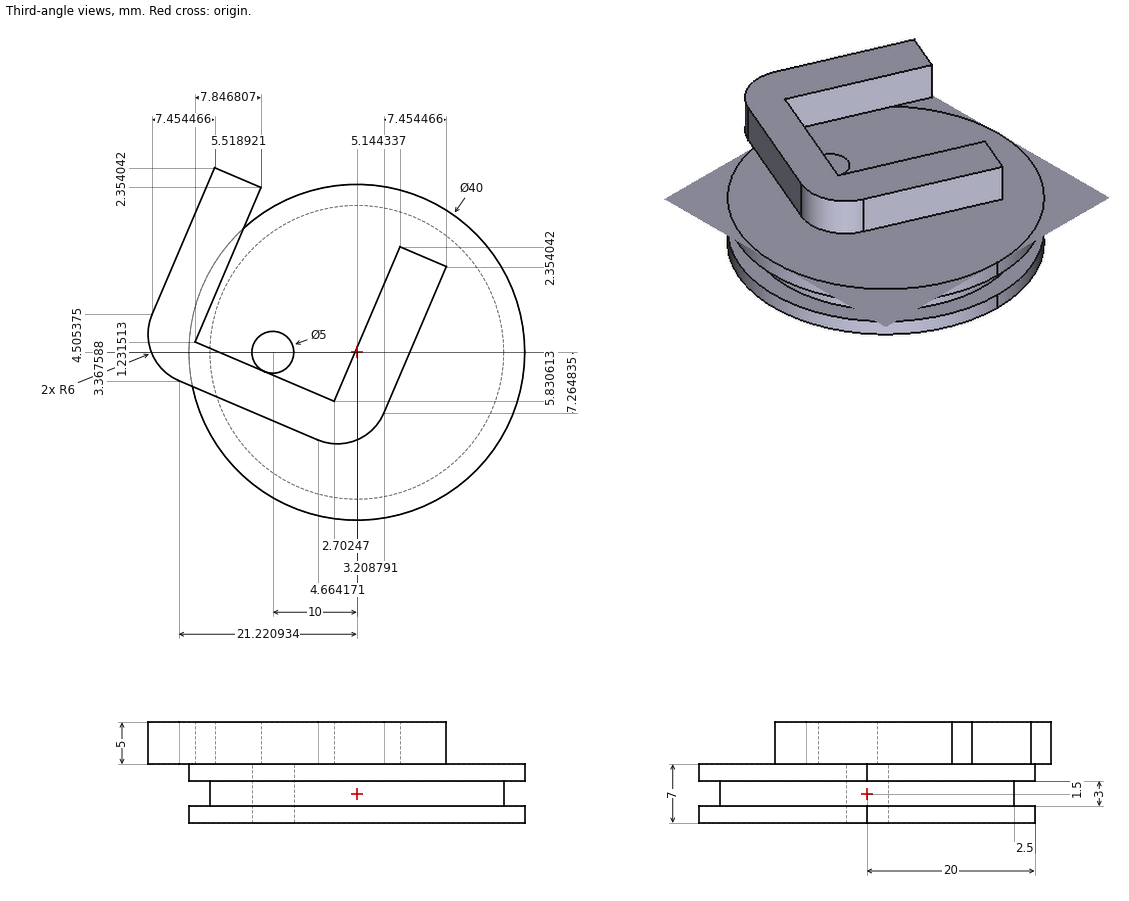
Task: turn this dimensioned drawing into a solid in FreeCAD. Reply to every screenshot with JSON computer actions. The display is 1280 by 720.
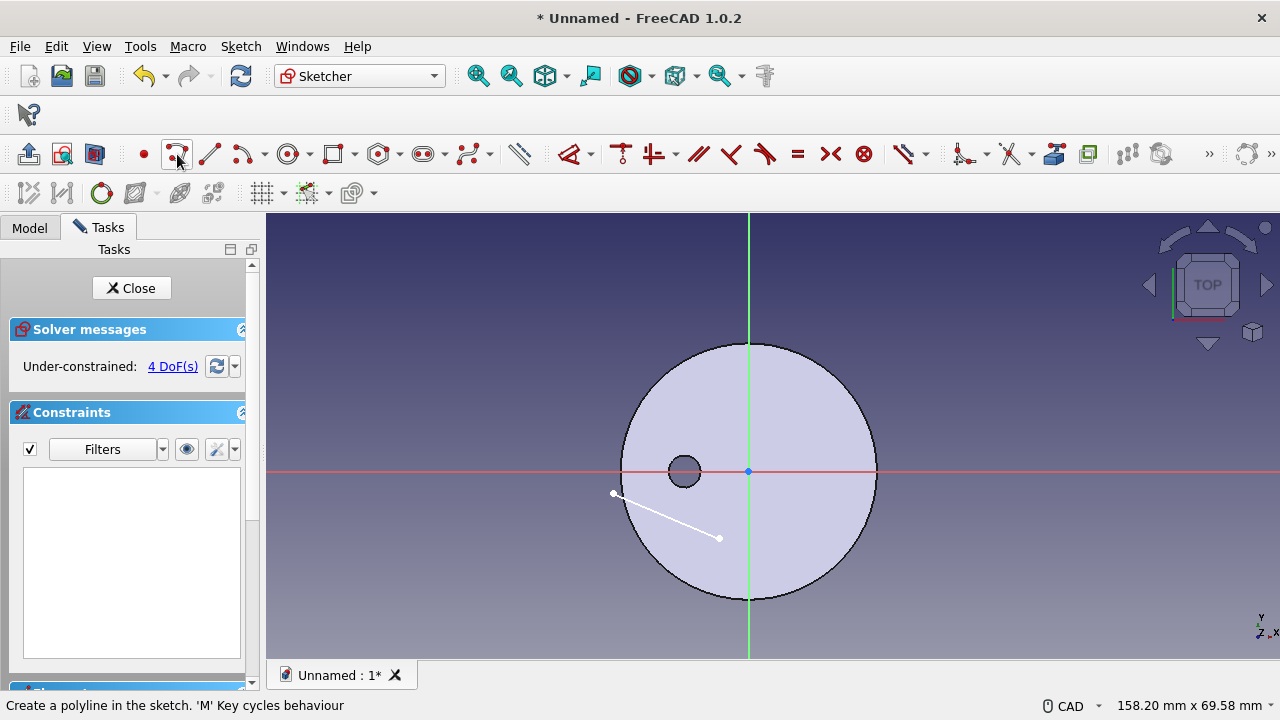
{"action": "left_click", "coordinate": [769, 518]}
{"action": "left_click", "coordinate": [817, 406]}
{"action": "left_click", "coordinate": [782, 391]}
{"action": "left_click", "coordinate": [731, 509]}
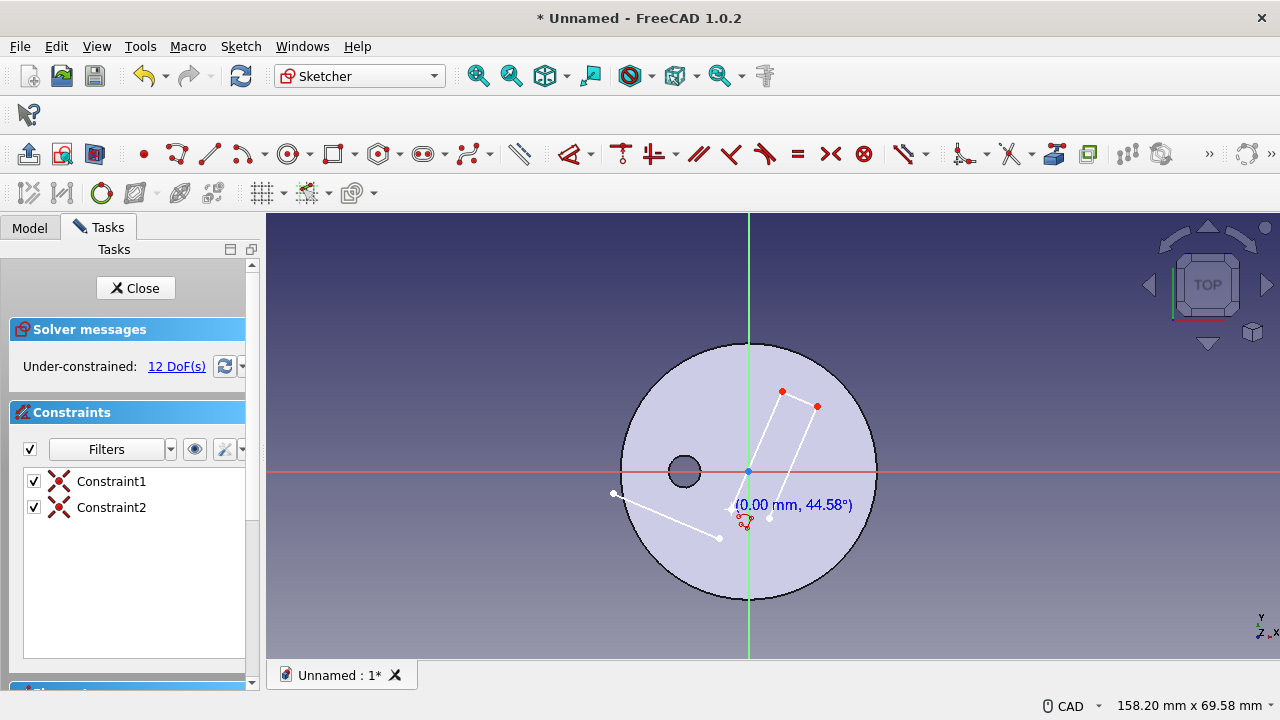
{"action": "scroll", "coordinate": [625, 464], "scroll_direction": "up", "scroll_amount": 4}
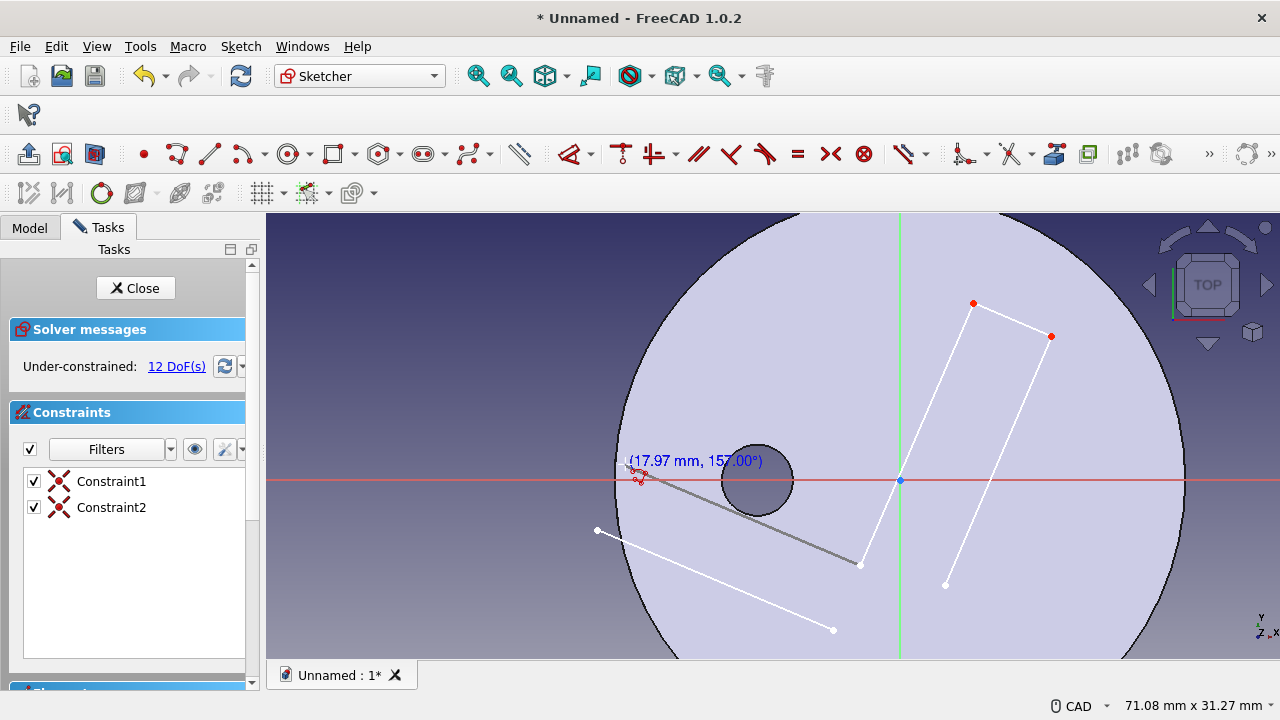
{"action": "left_click", "coordinate": [625, 463]}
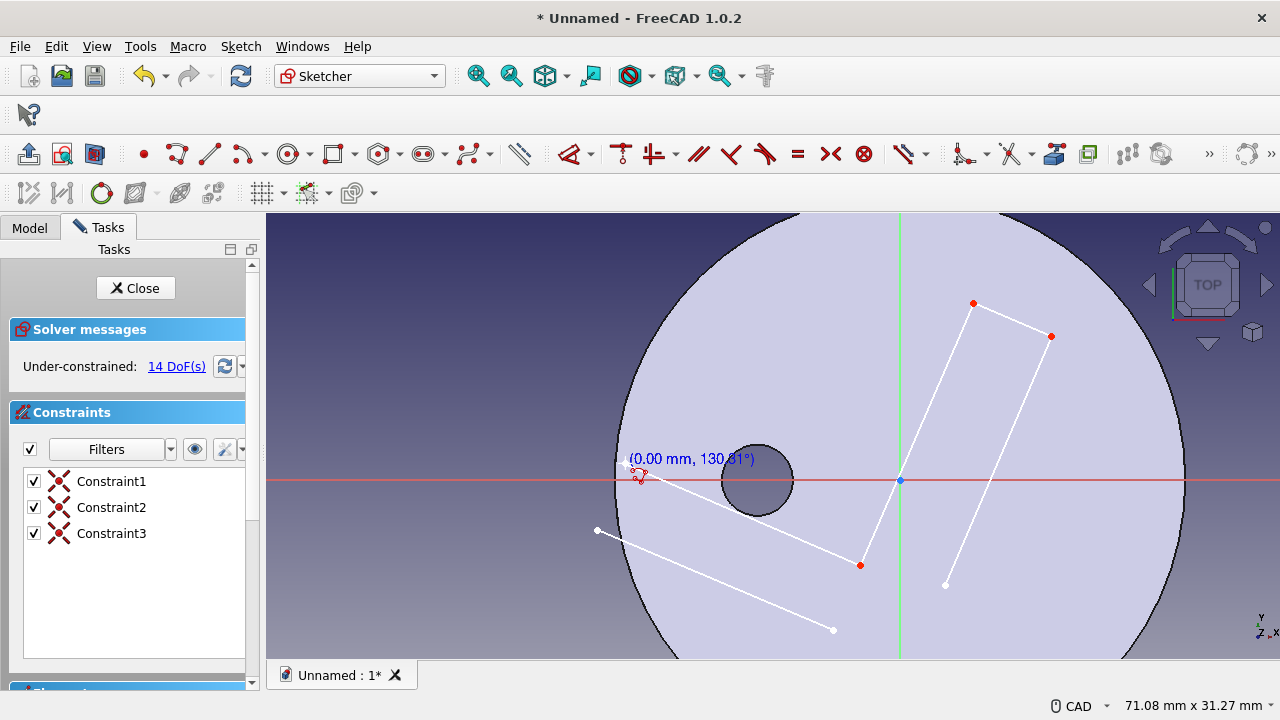
{"action": "scroll", "coordinate": [586, 482], "scroll_direction": "down", "scroll_amount": 3}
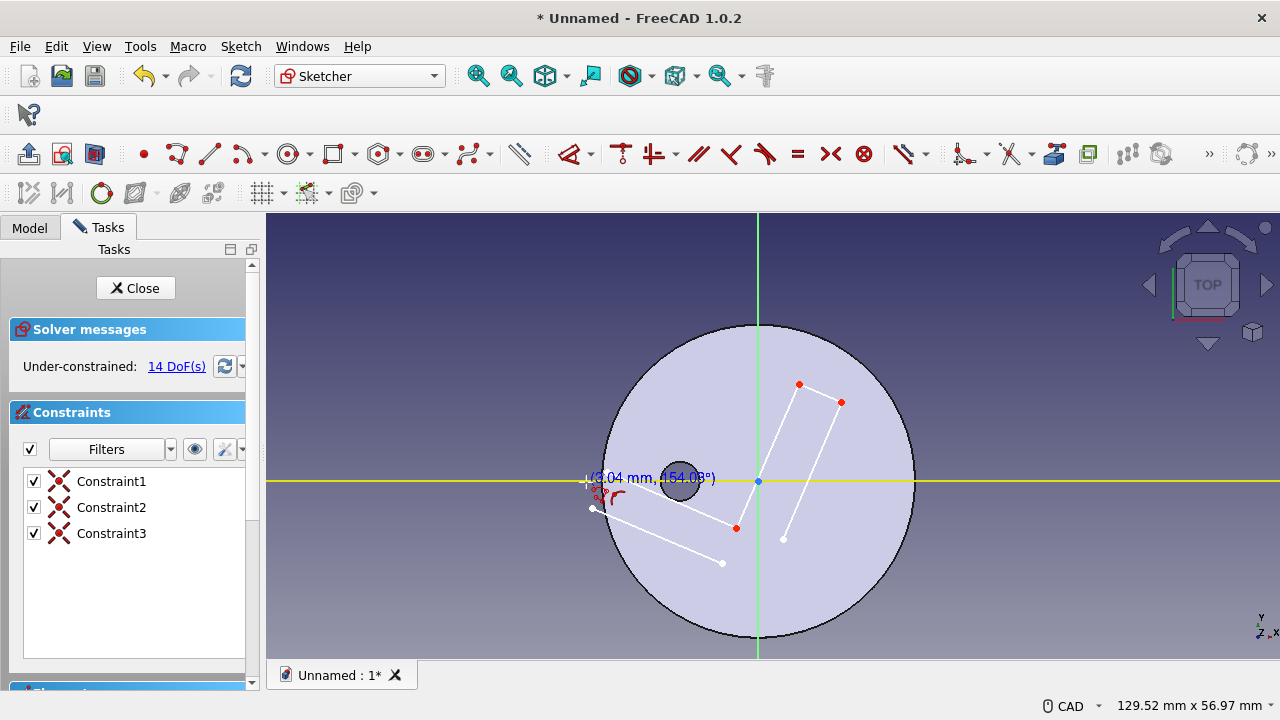
{"action": "left_click", "coordinate": [669, 328]}
{"action": "left_click", "coordinate": [626, 309]}
{"action": "left_click", "coordinate": [568, 446]}
{"action": "right_click", "coordinate": [568, 446]}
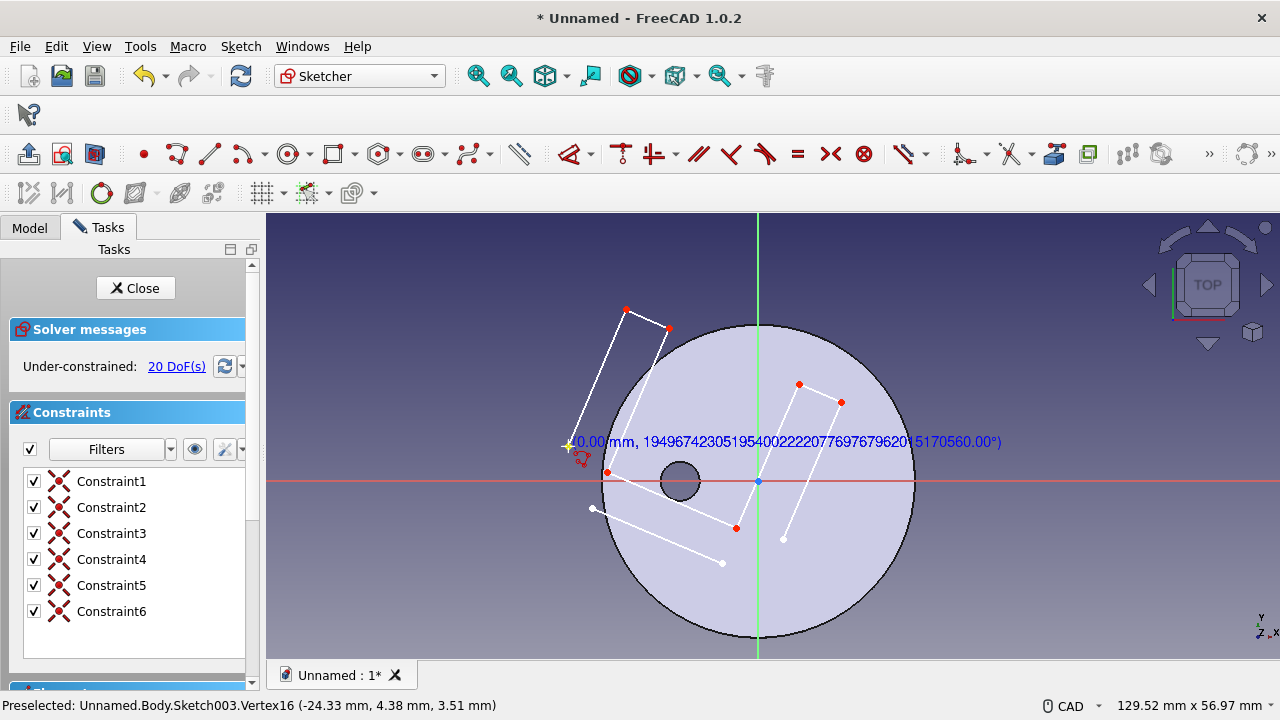
{"action": "left_click", "coordinate": [264, 154]}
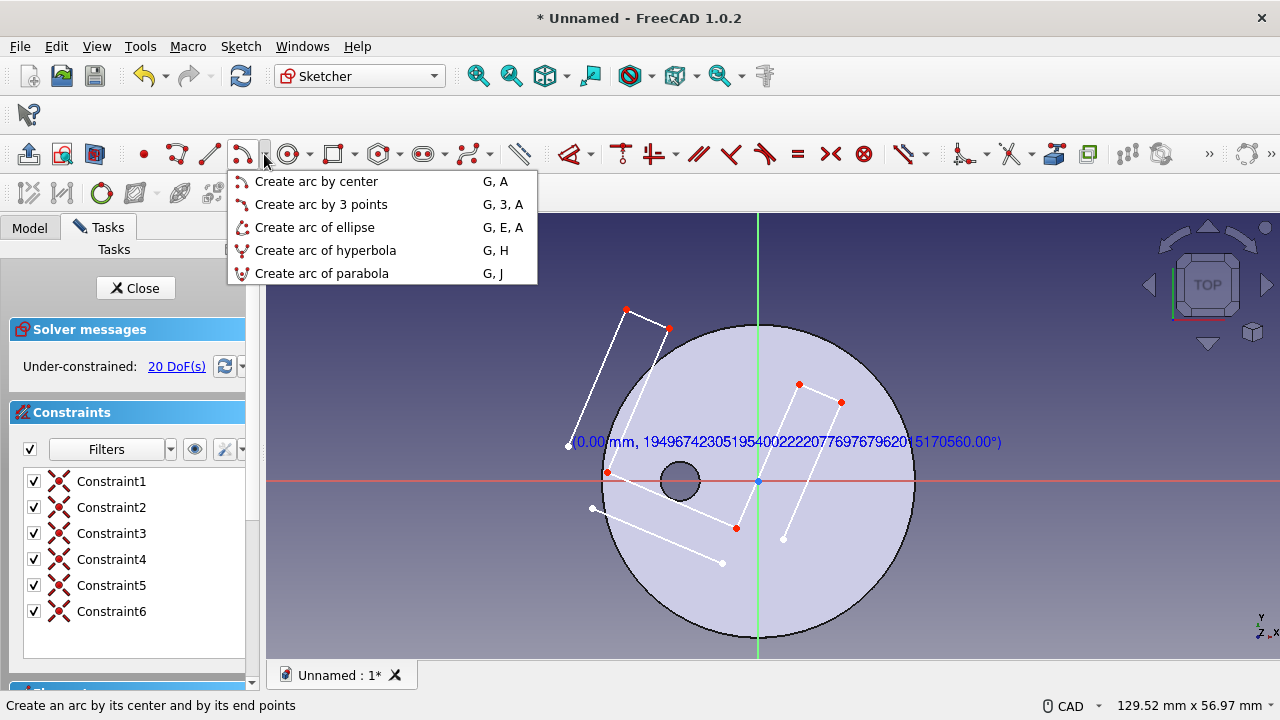
{"action": "left_click", "coordinate": [382, 204]}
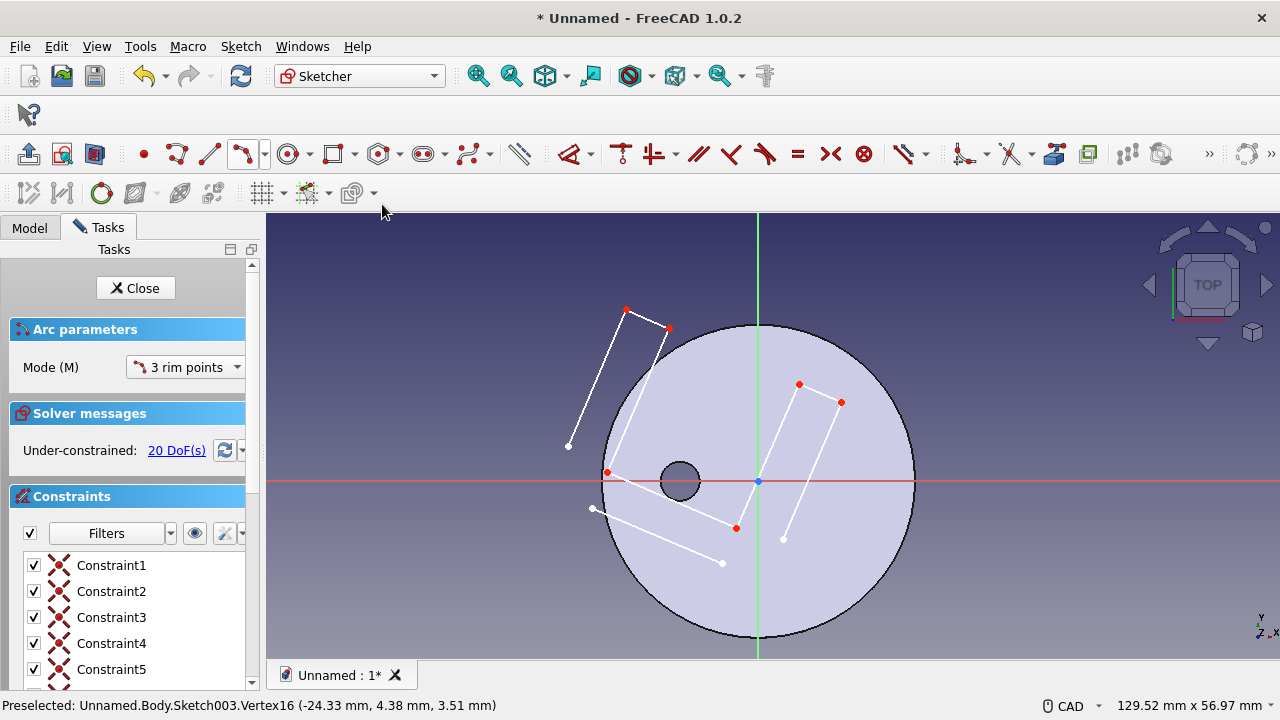
{"action": "left_click", "coordinate": [722, 564]}
{"action": "left_click", "coordinate": [783, 539]}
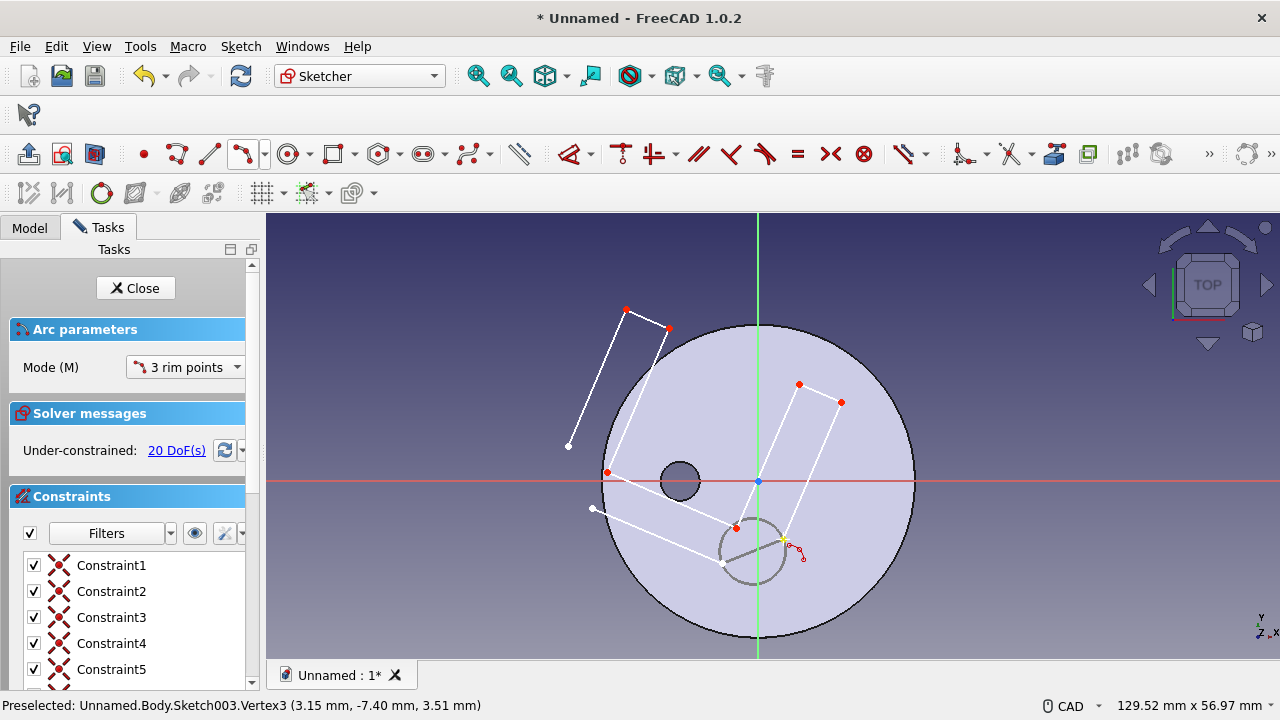
{"action": "scroll", "coordinate": [744, 567], "scroll_direction": "up", "scroll_amount": 2}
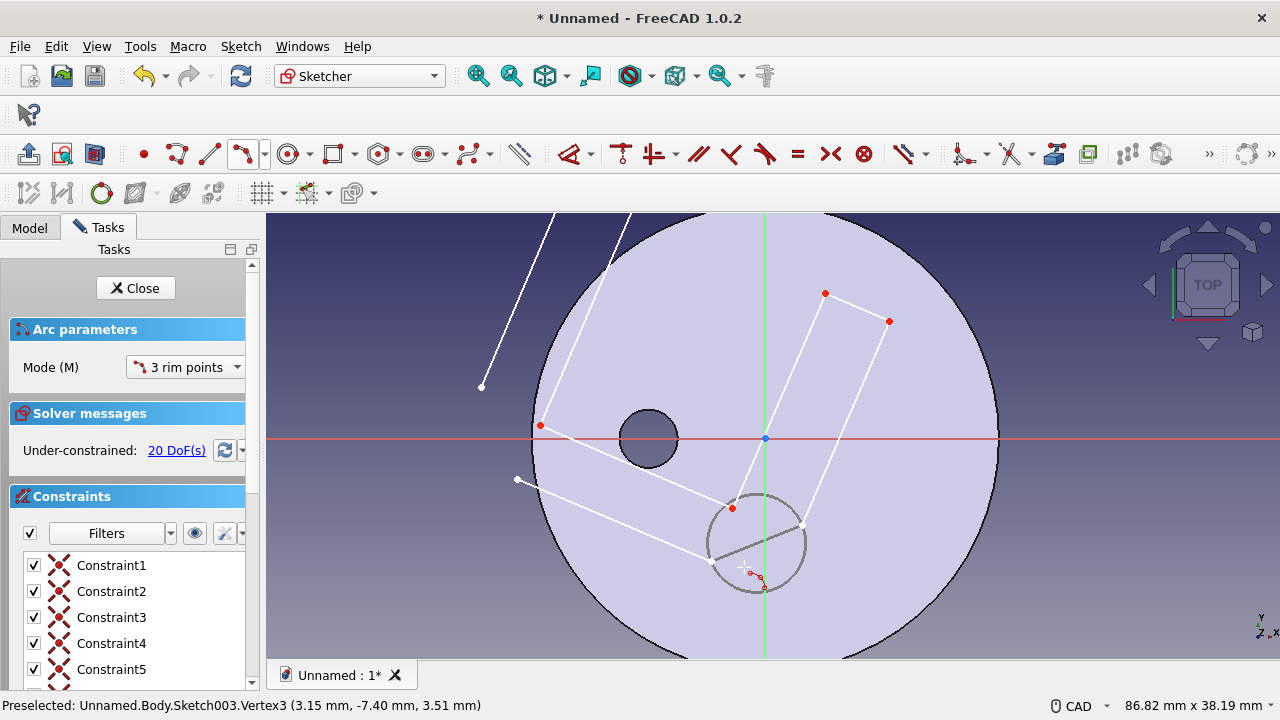
{"action": "left_click", "coordinate": [743, 566]}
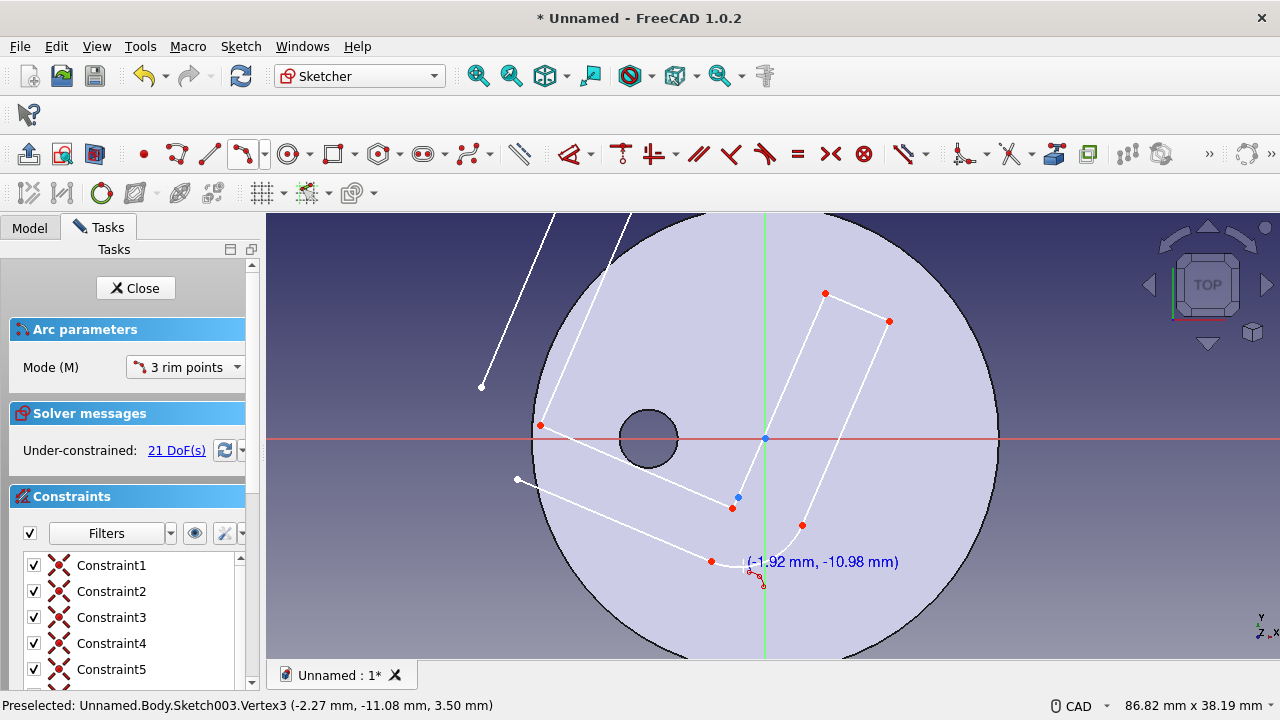
{"action": "left_click", "coordinate": [481, 388]}
{"action": "left_click", "coordinate": [518, 480]}
{"action": "left_click", "coordinate": [491, 459]}
{"action": "key", "text": "Escape"}